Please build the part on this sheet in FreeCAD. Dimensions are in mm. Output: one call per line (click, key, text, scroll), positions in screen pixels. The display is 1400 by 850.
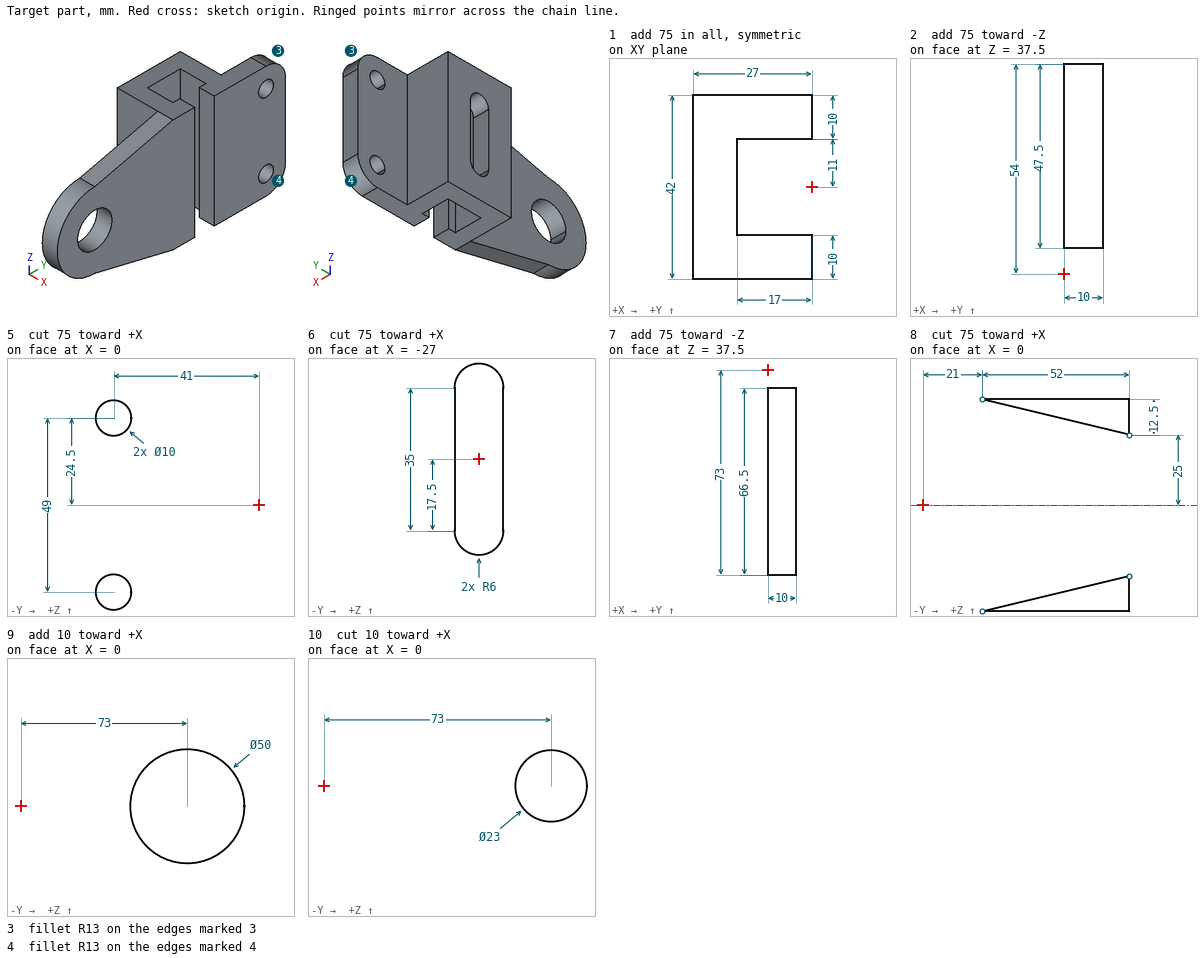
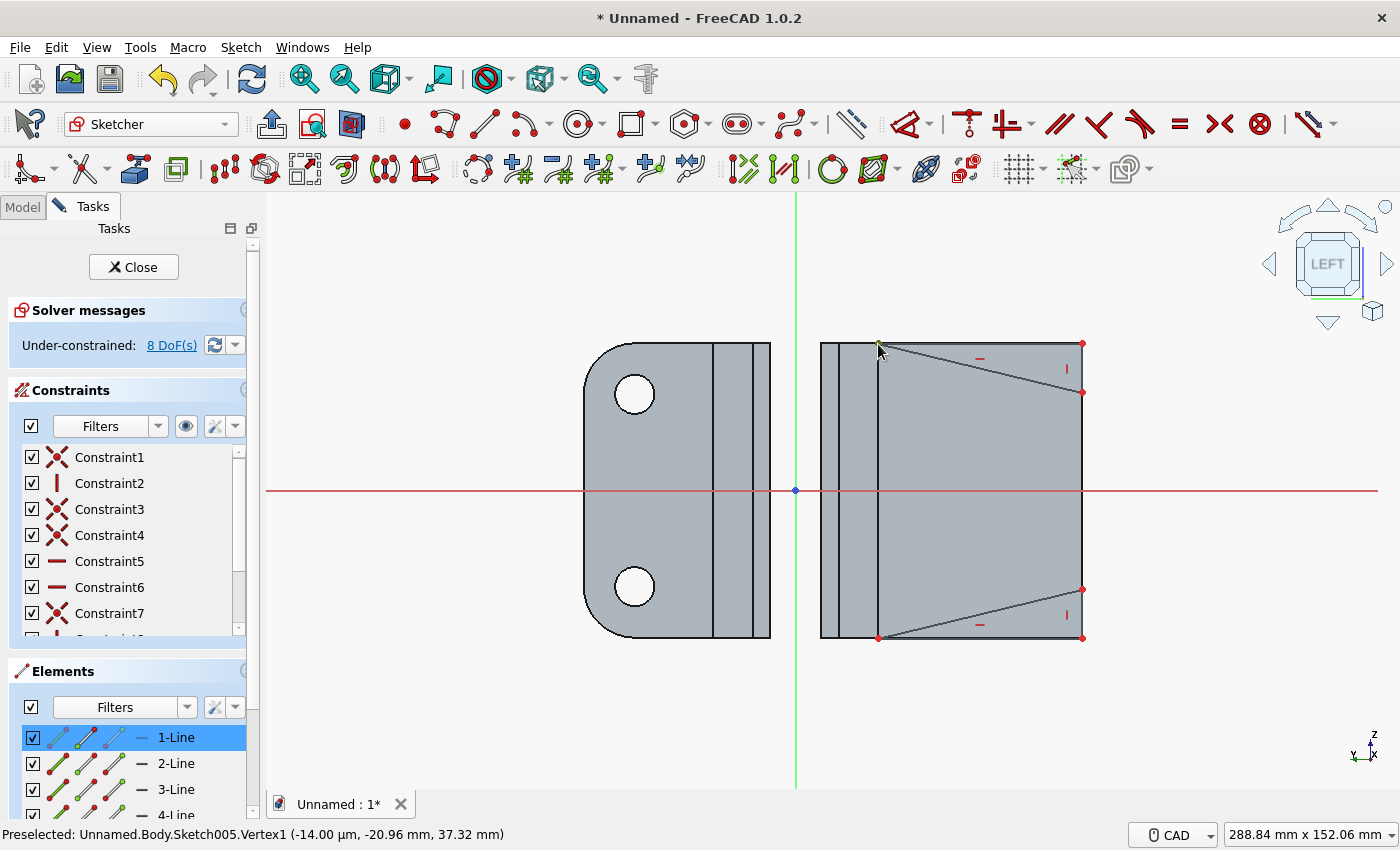
click(878, 639)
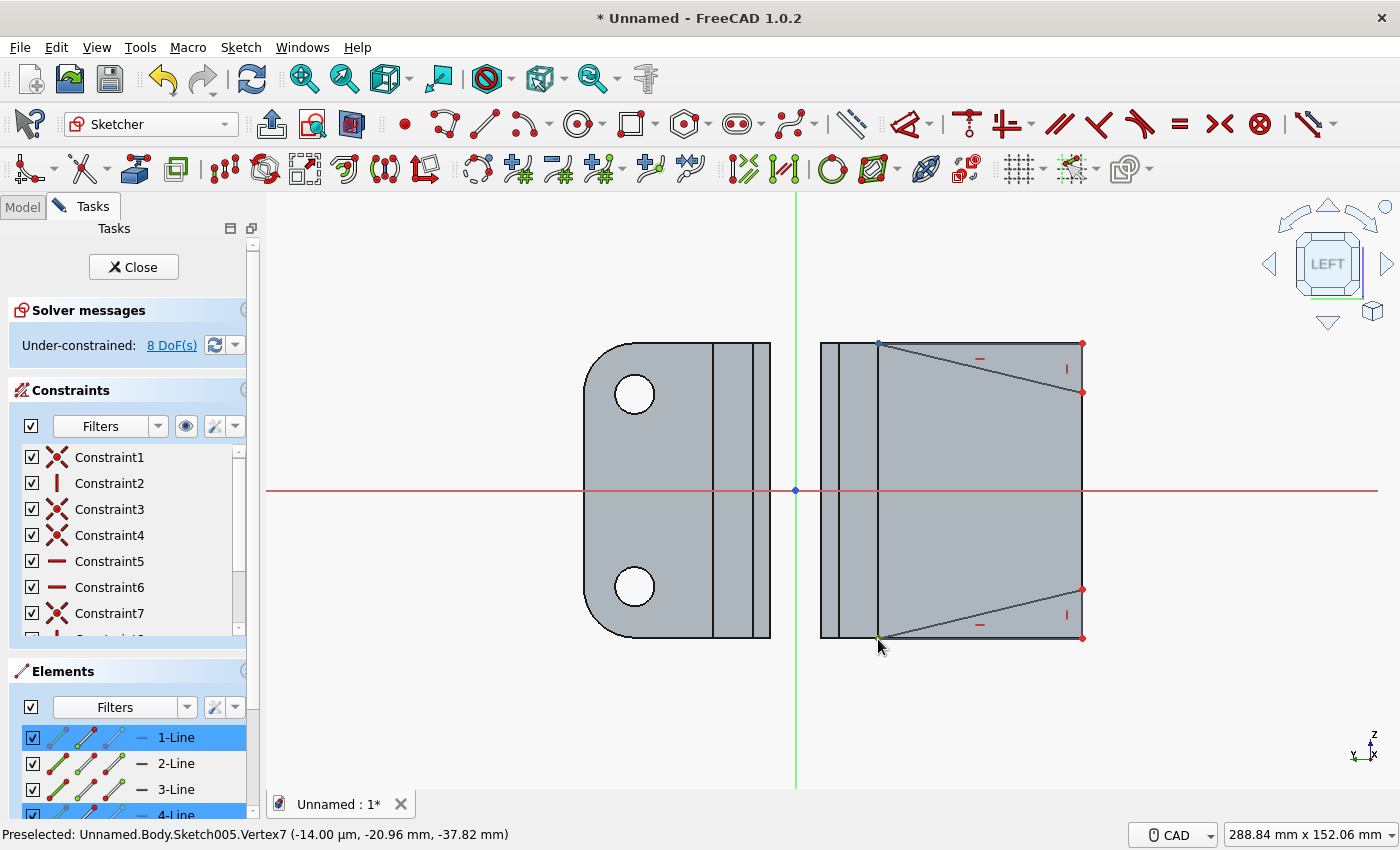
click(361, 490)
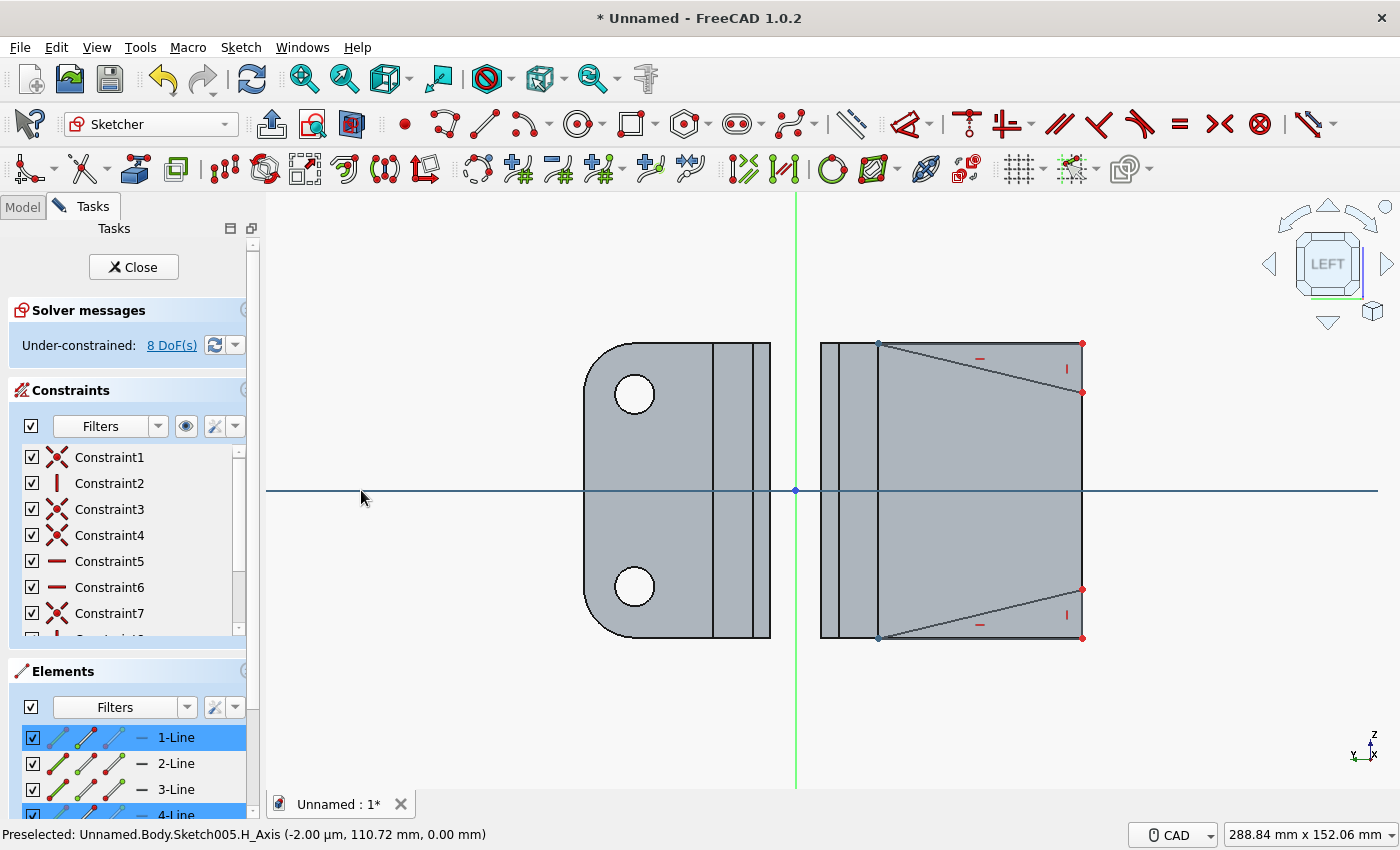
key(s)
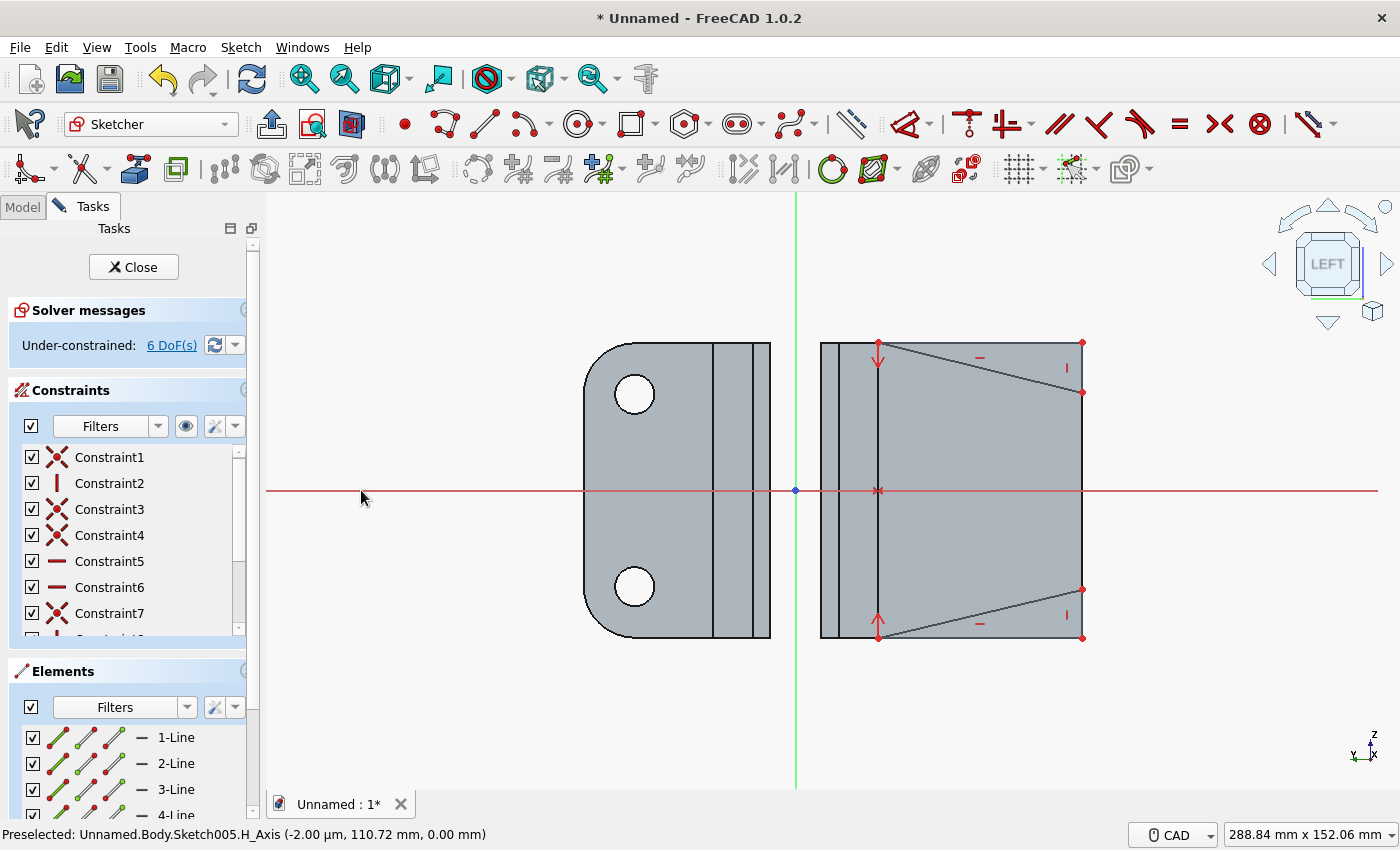
click(1082, 393)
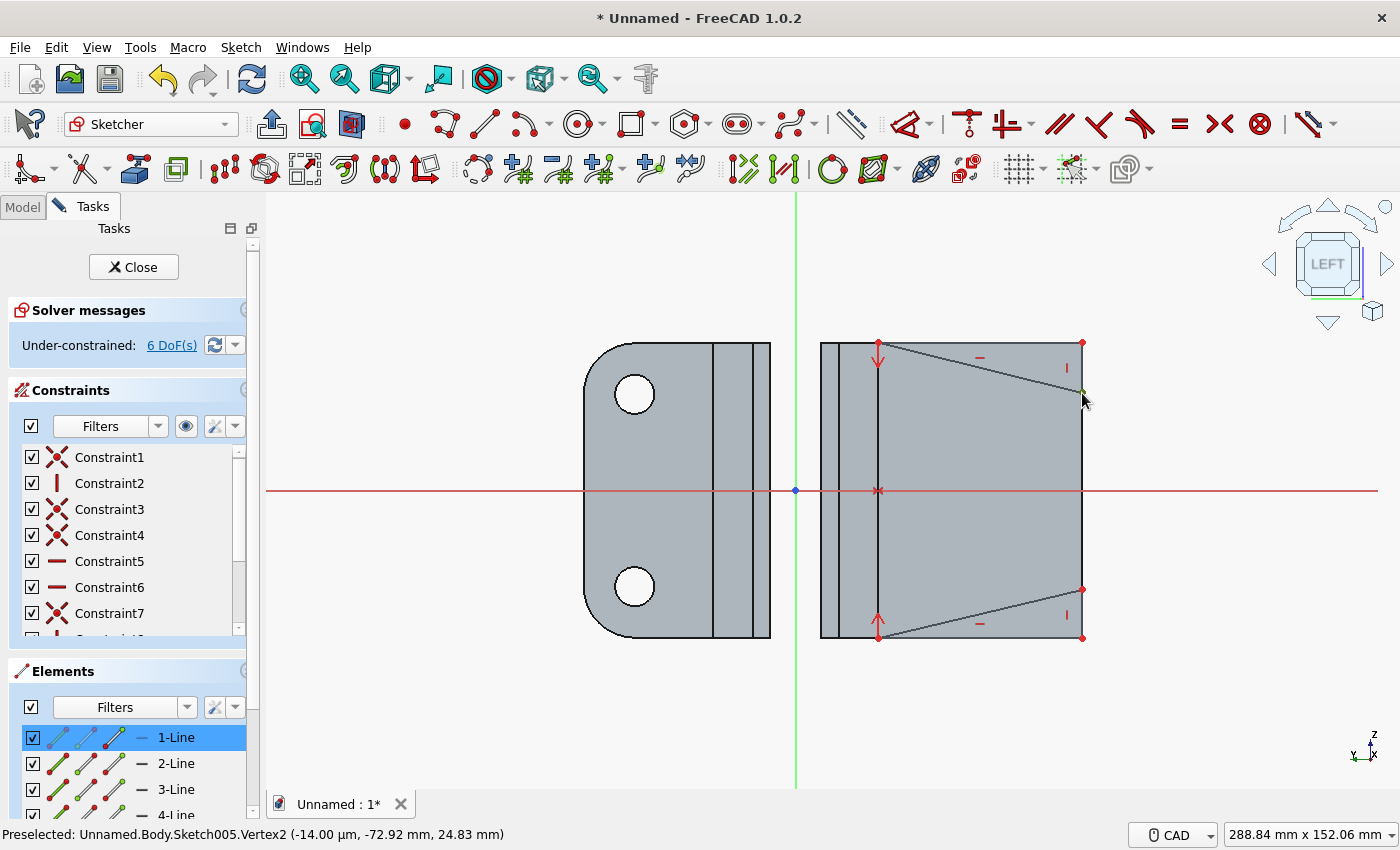
click(1082, 590)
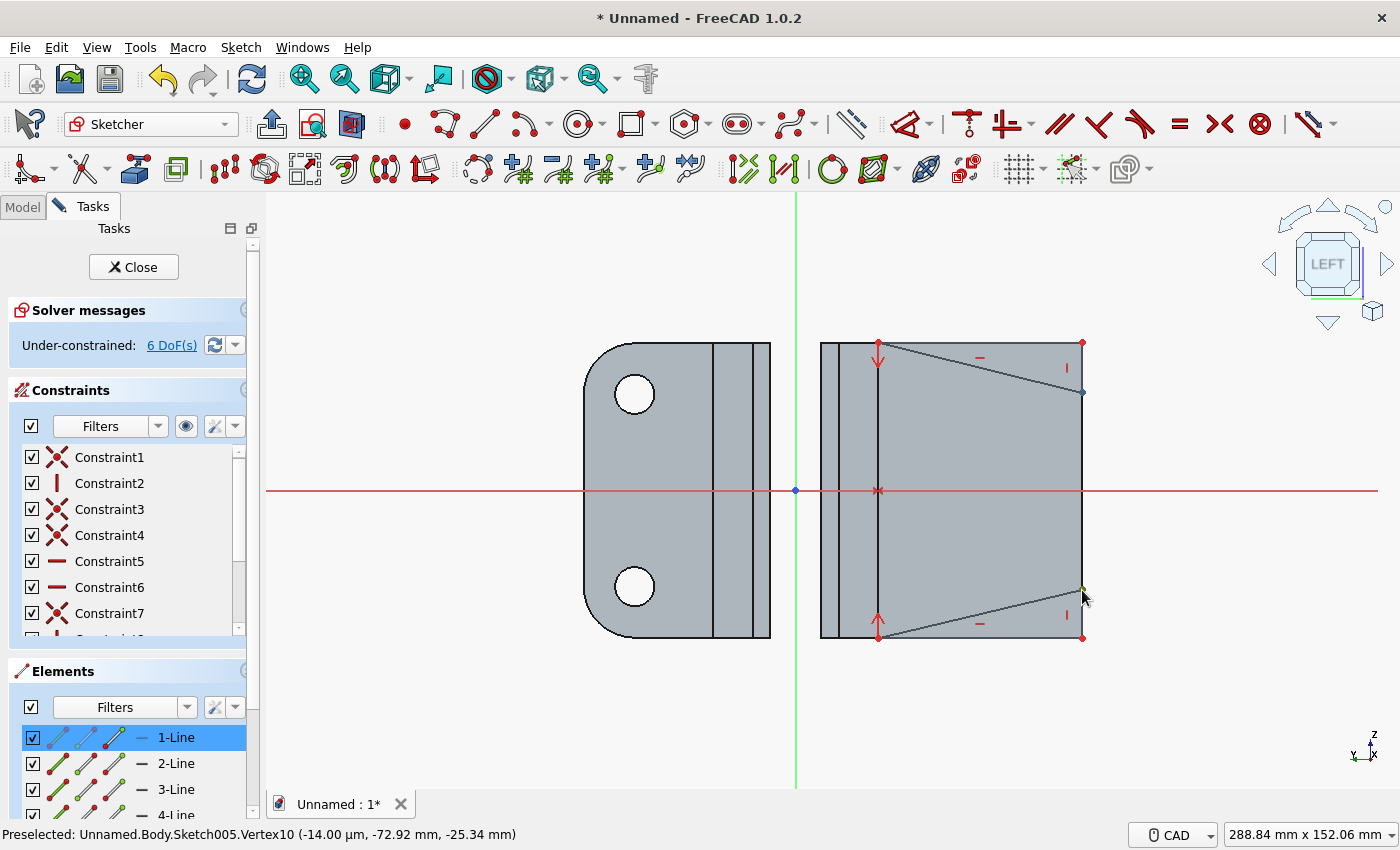
click(361, 490)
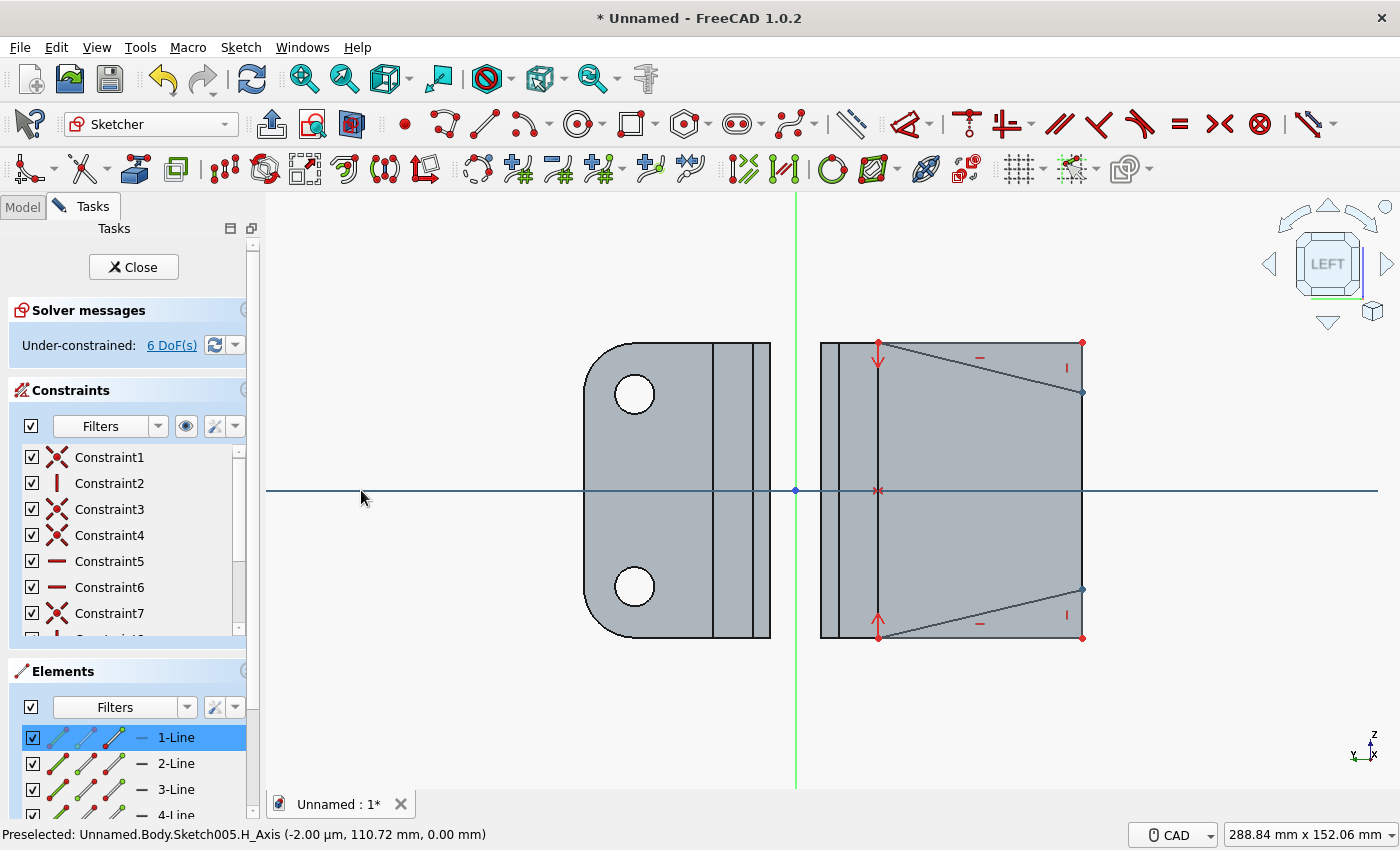
key(s)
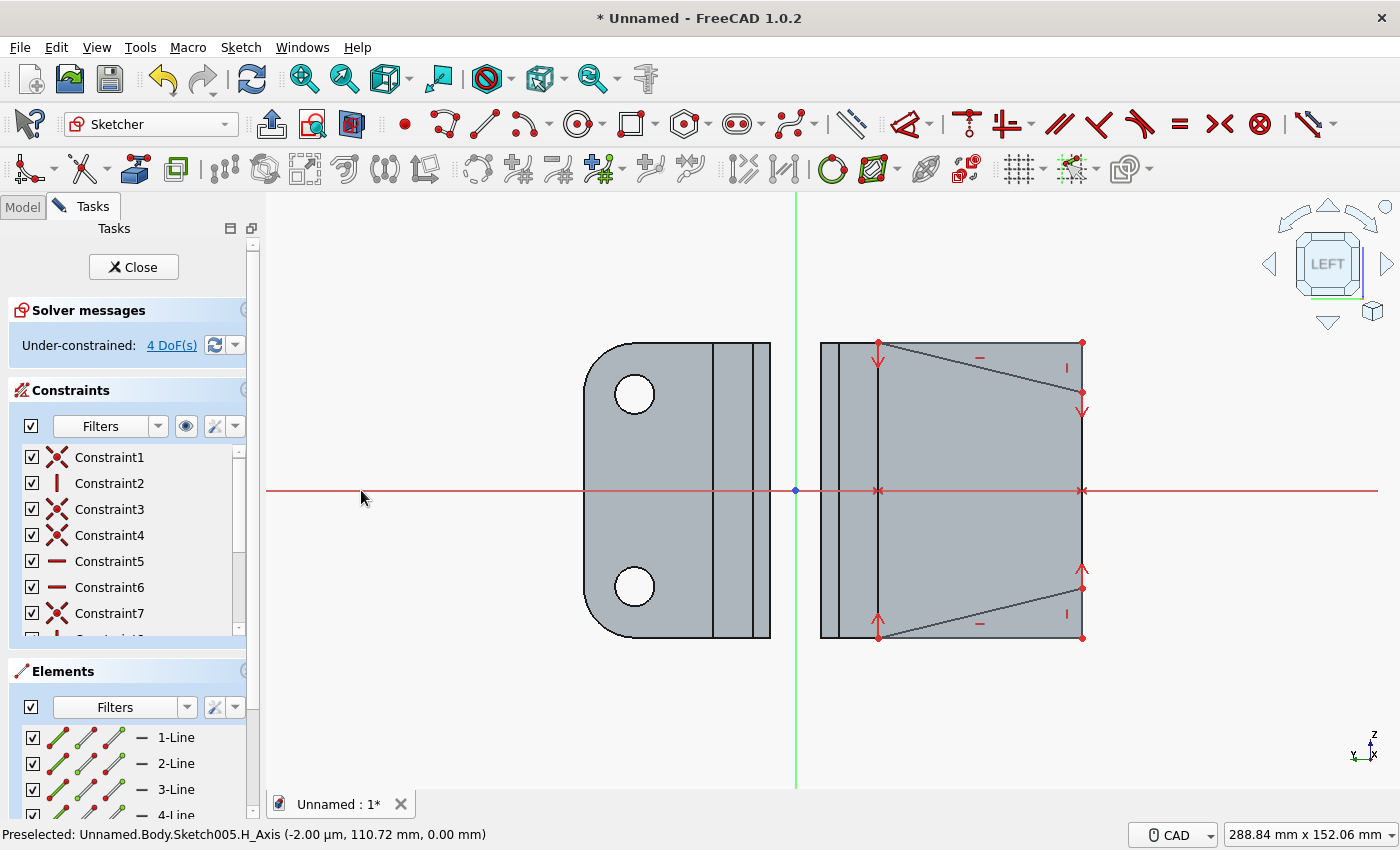
key(d)